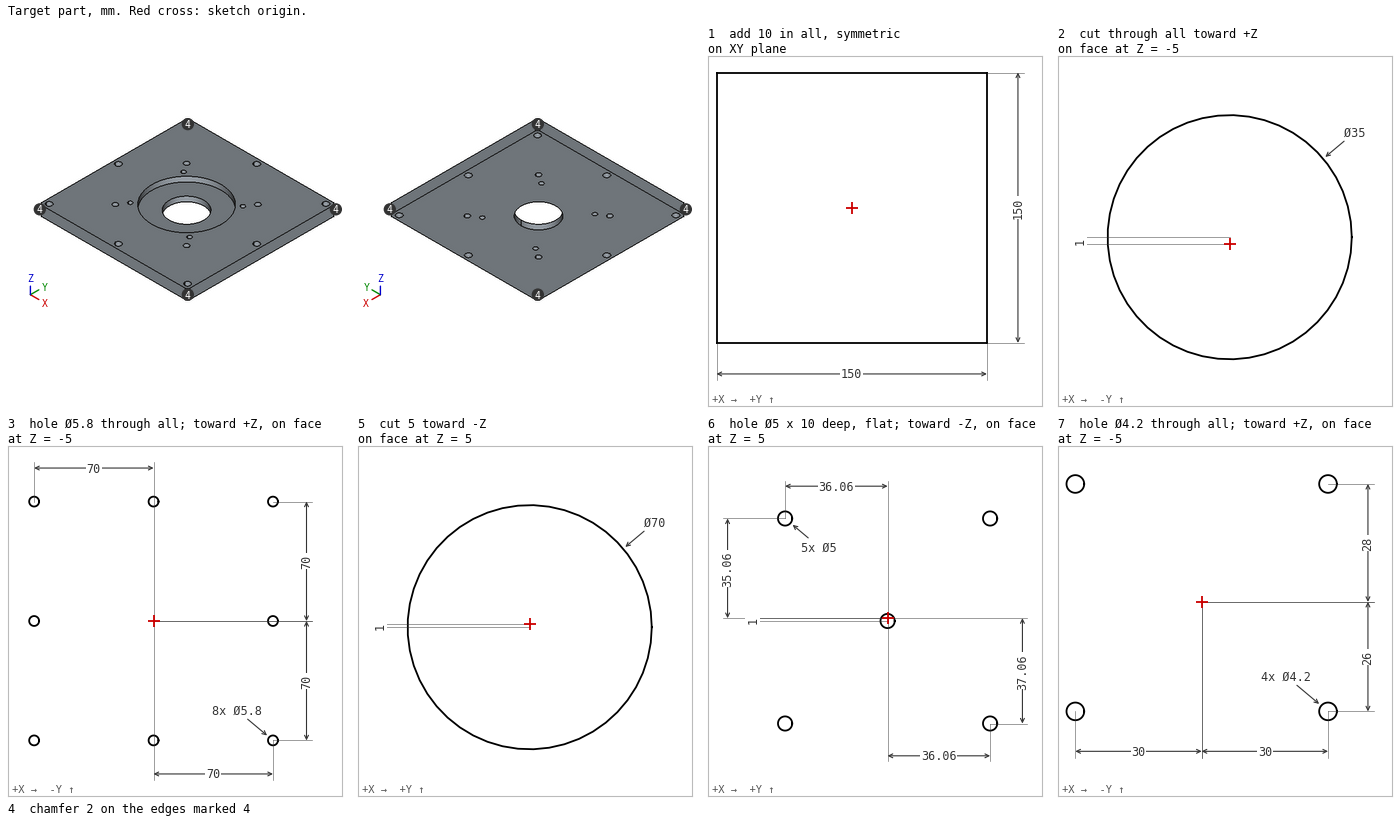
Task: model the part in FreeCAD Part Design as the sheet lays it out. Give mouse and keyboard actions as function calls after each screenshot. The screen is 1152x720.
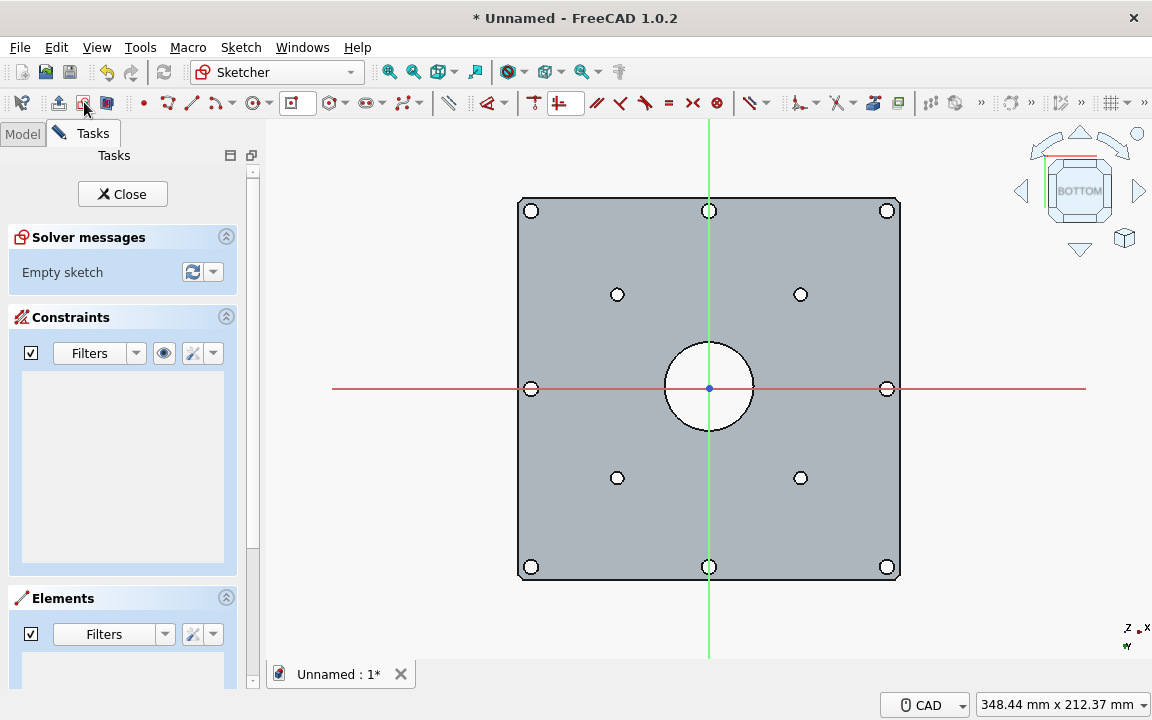
scroll(765, 384, up, 4)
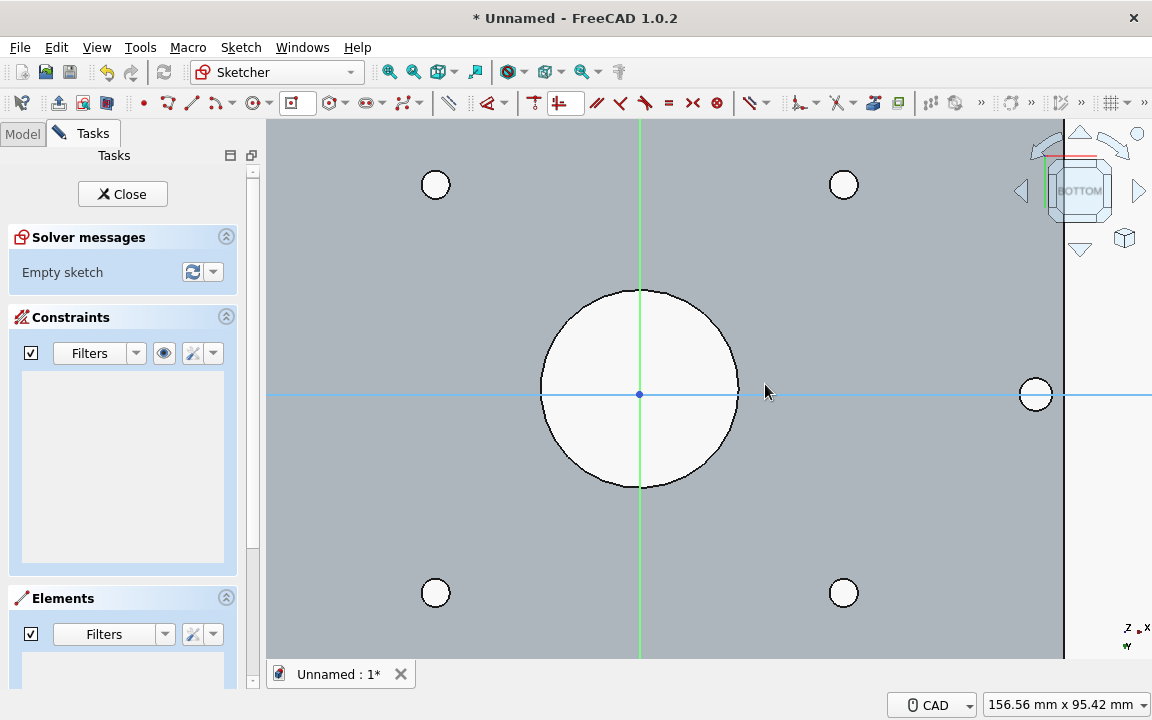
click(254, 104)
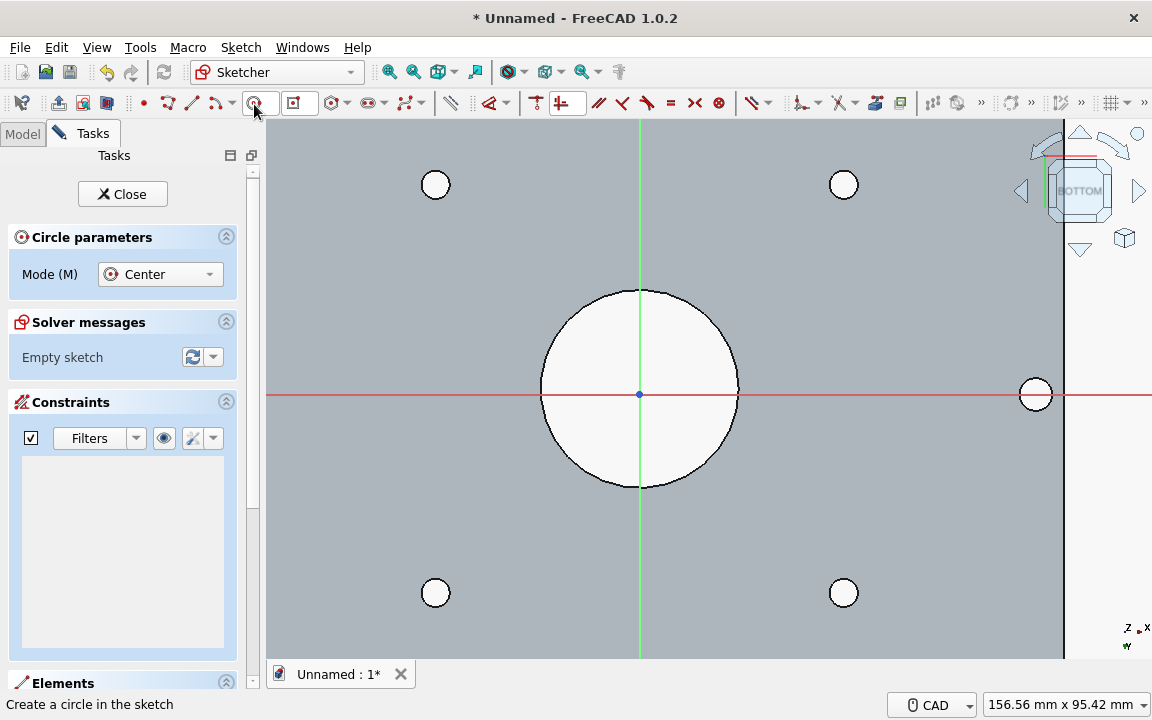
scroll(809, 542, up, 4)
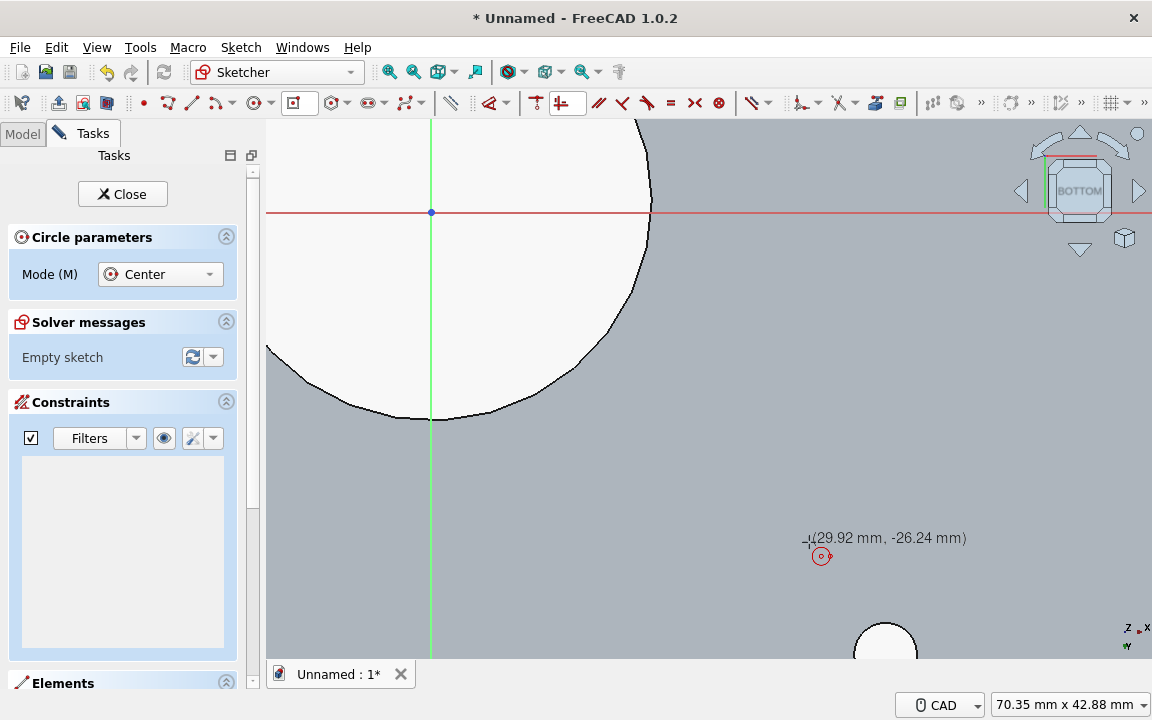
click(809, 540)
move(828, 522)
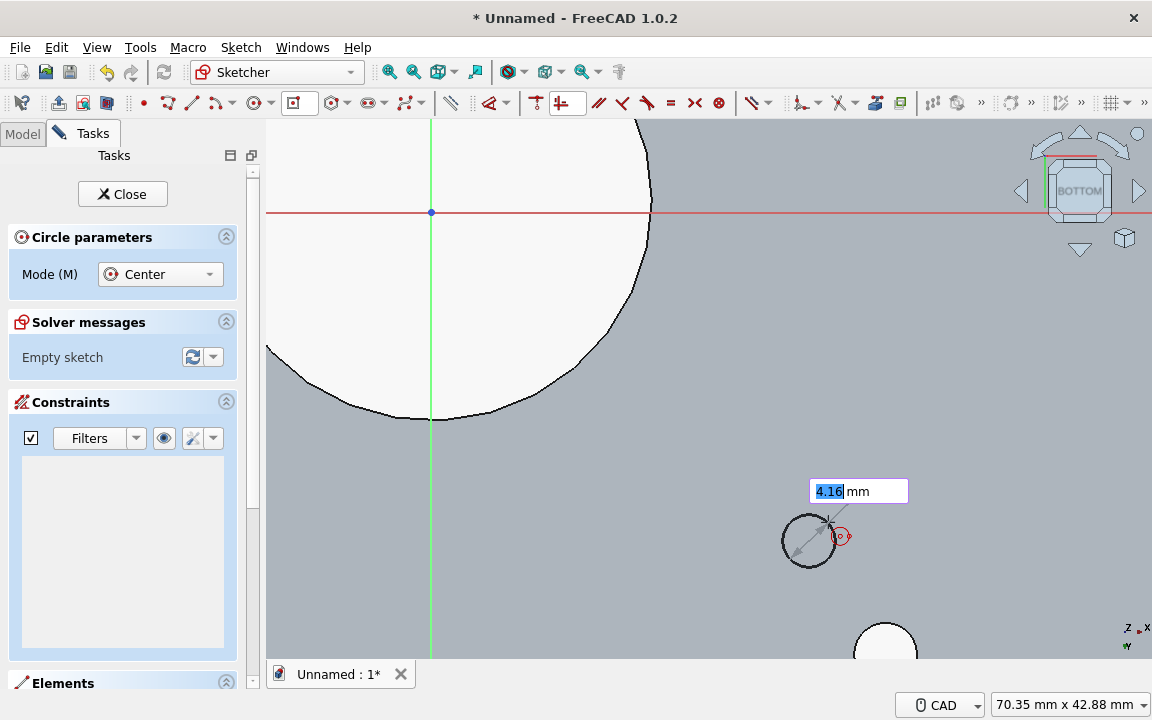
text(4.2)
key(Return)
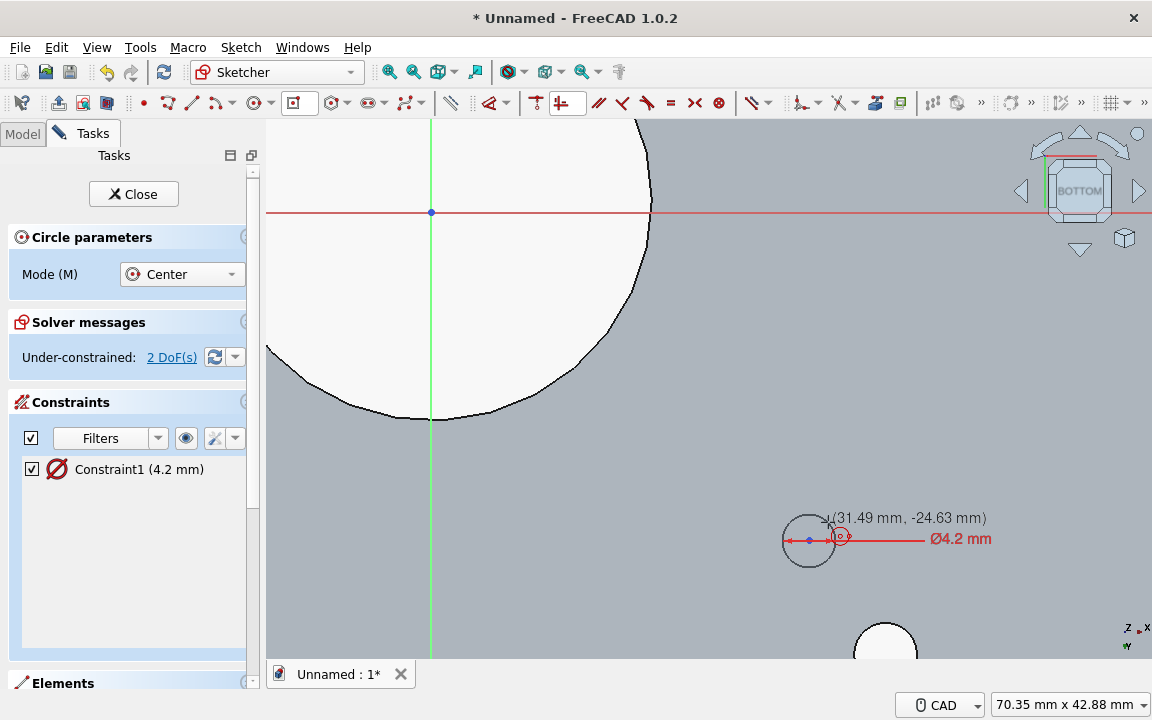
scroll(811, 543, down, 4)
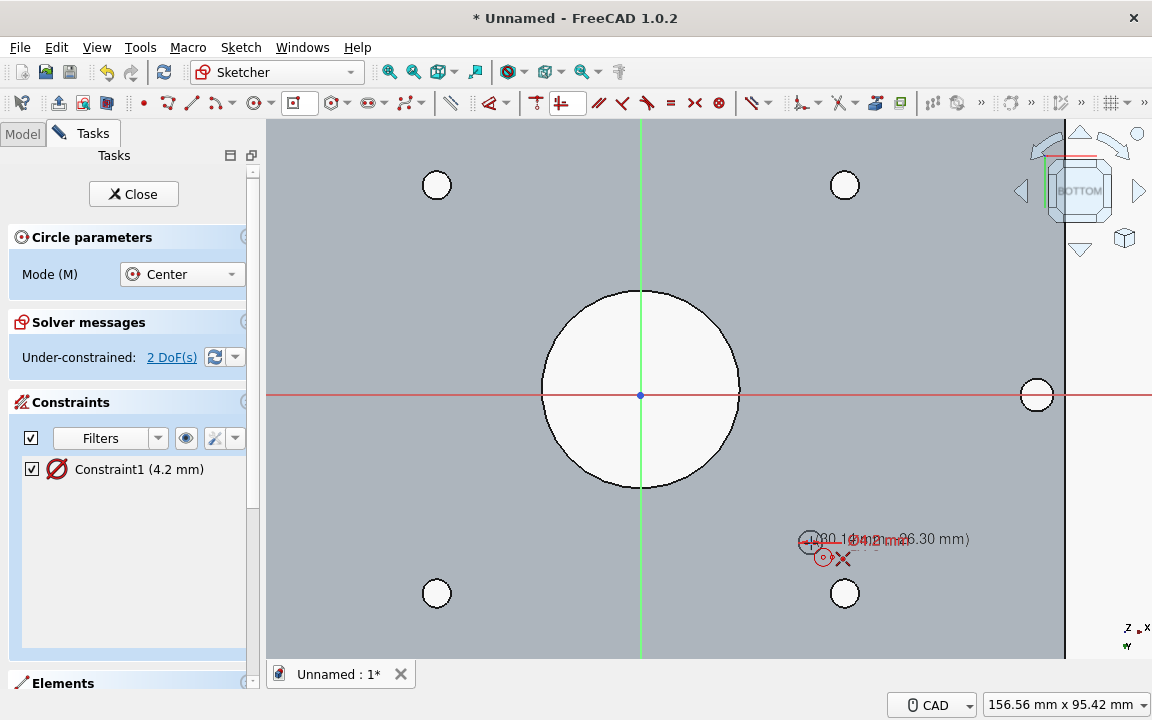
scroll(471, 542, up, 4)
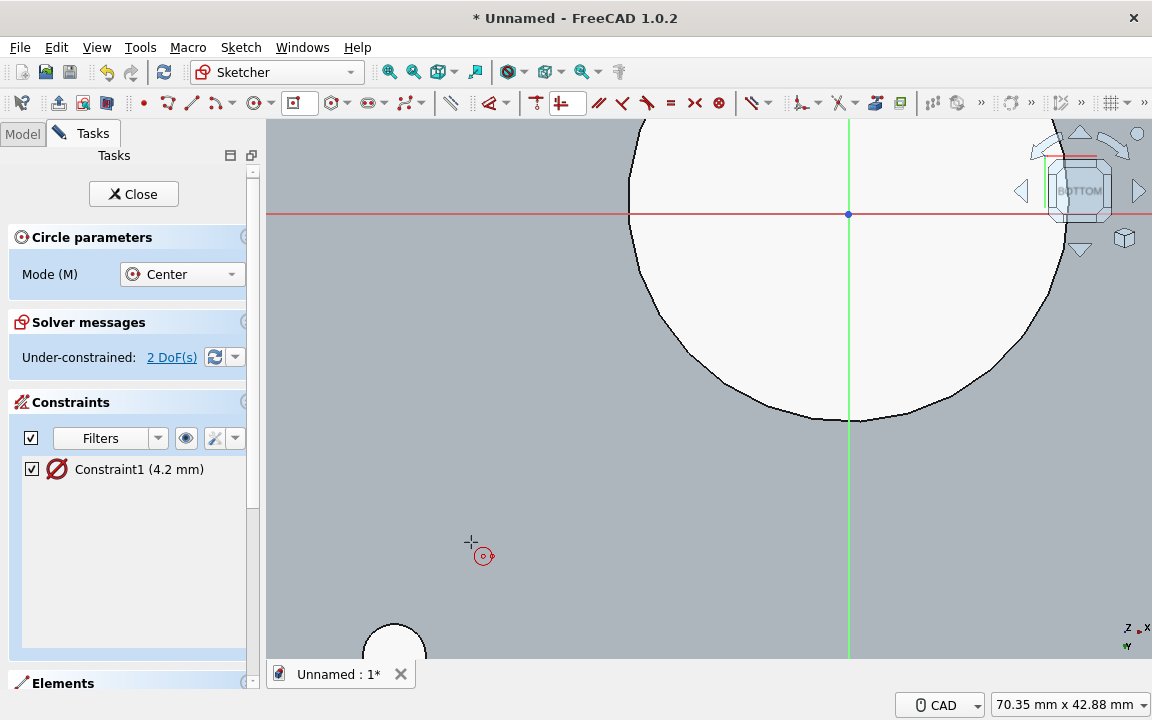
click(471, 542)
move(489, 523)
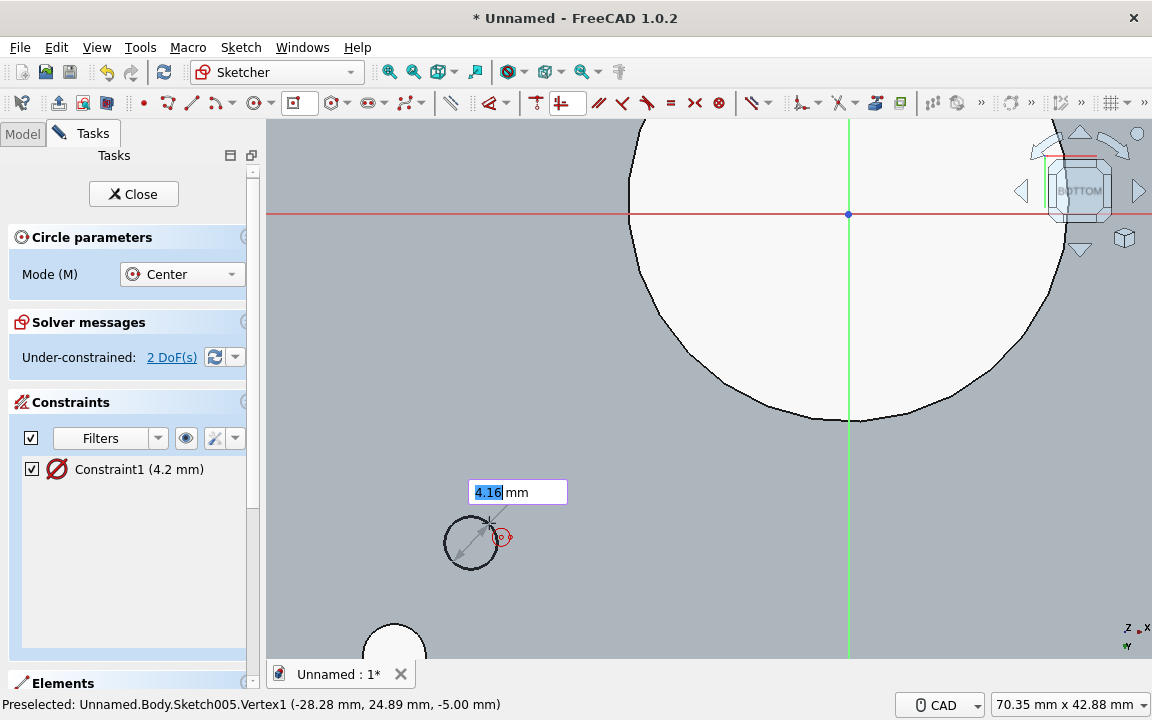
text(4.2)
key(Return)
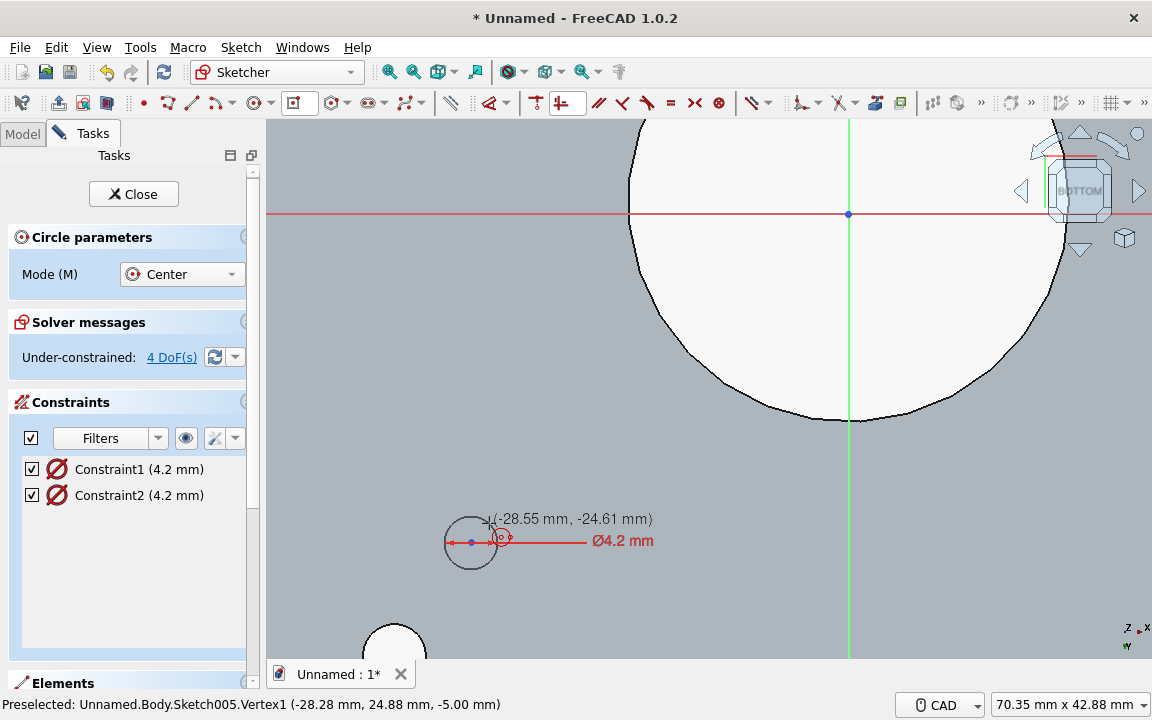
scroll(471, 542, down, 4)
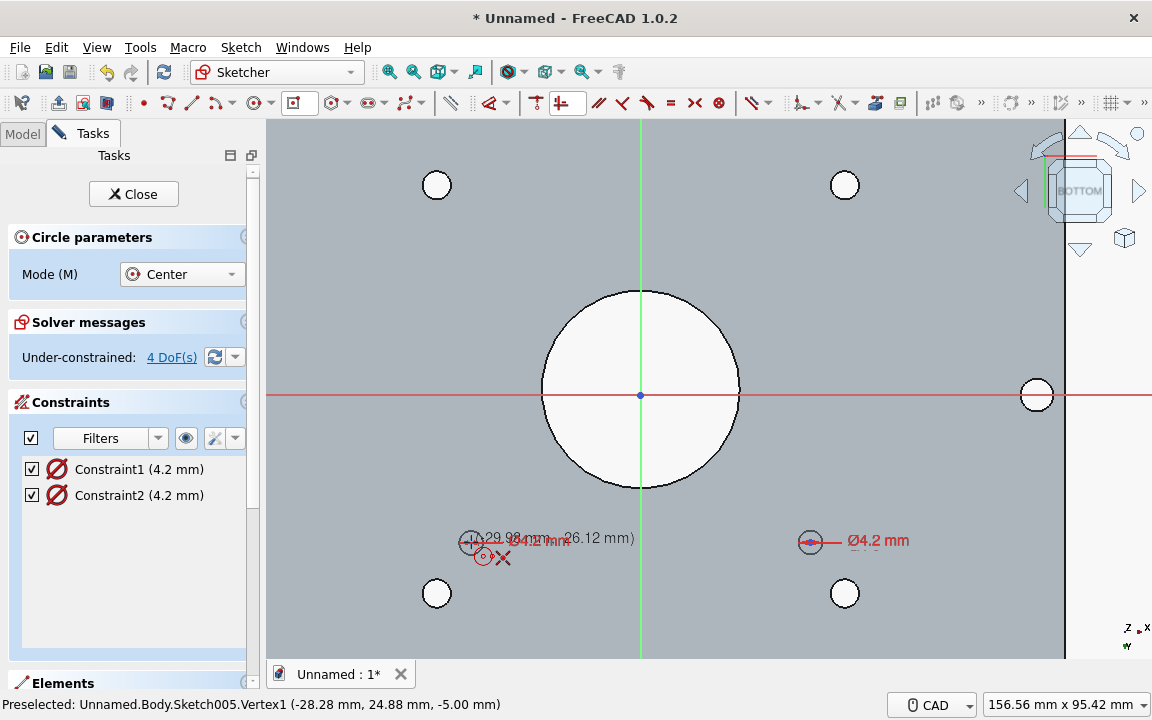
scroll(811, 237, up, 4)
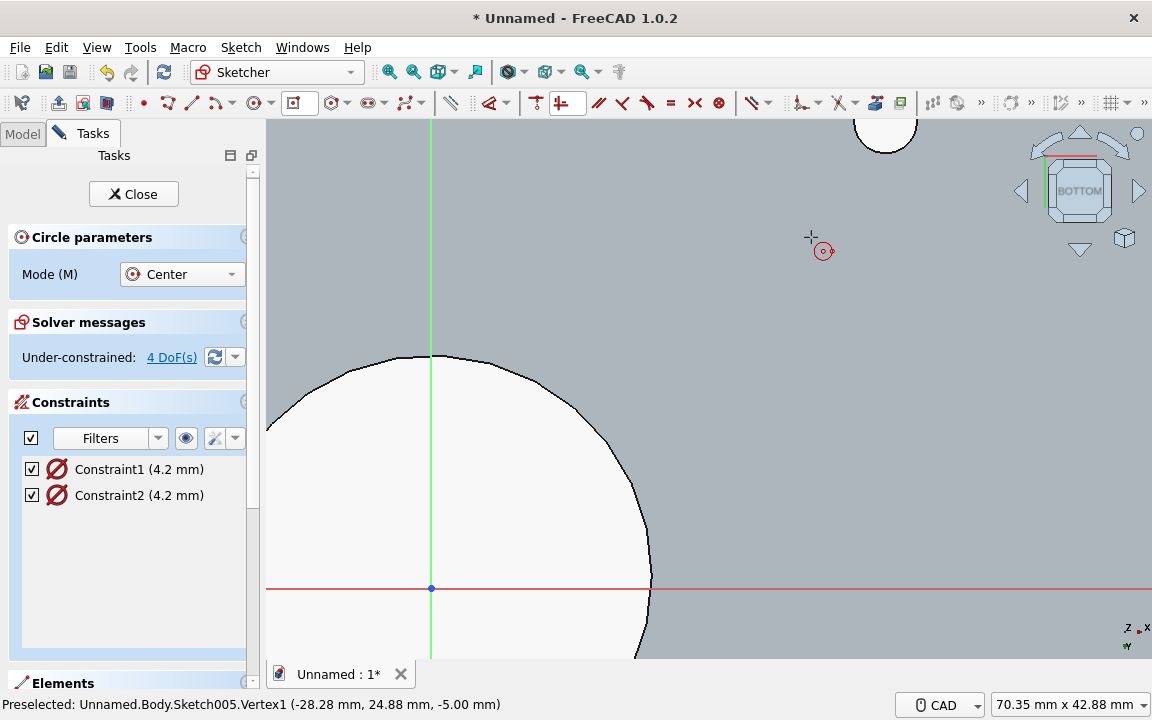
click(809, 236)
move(828, 217)